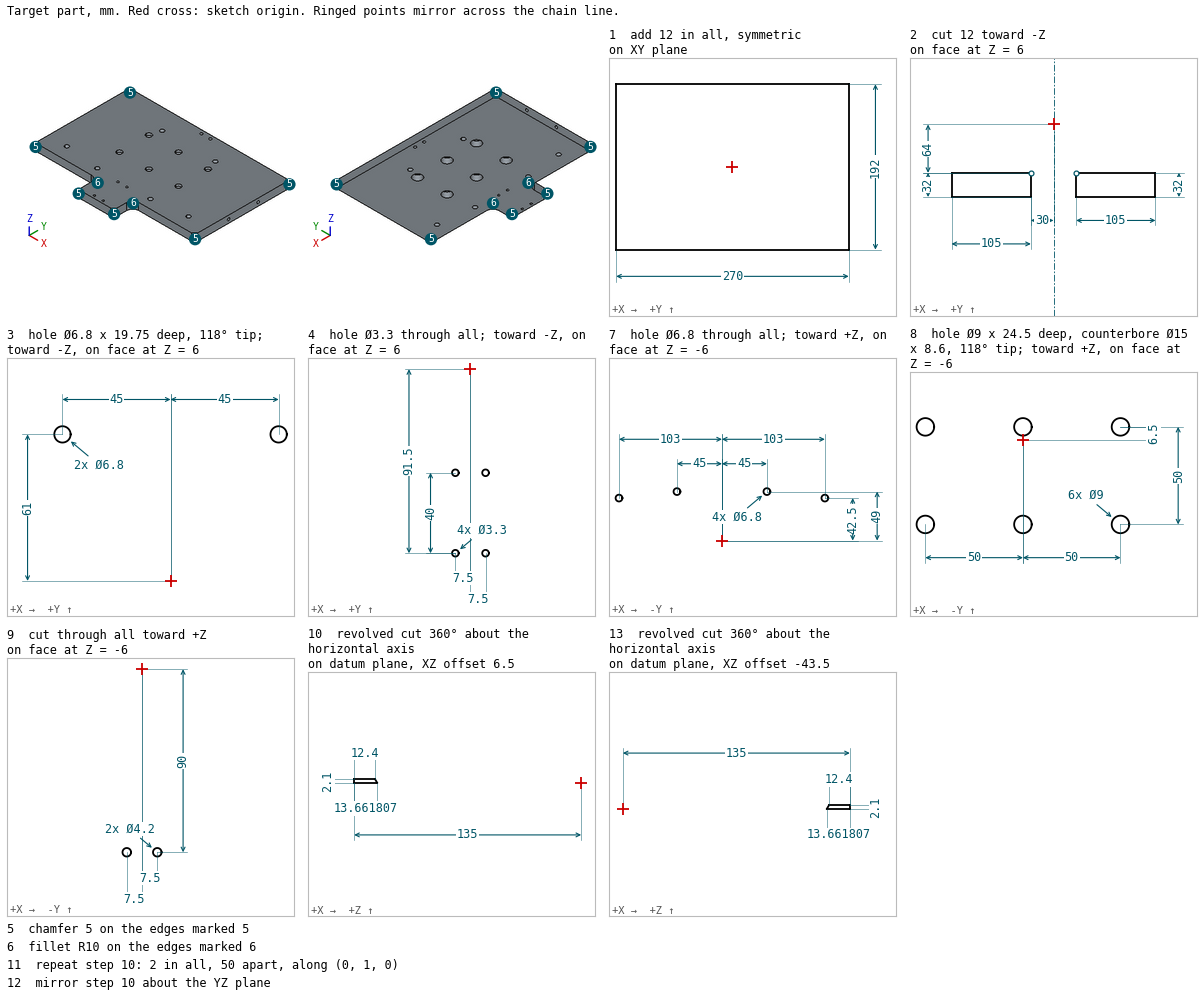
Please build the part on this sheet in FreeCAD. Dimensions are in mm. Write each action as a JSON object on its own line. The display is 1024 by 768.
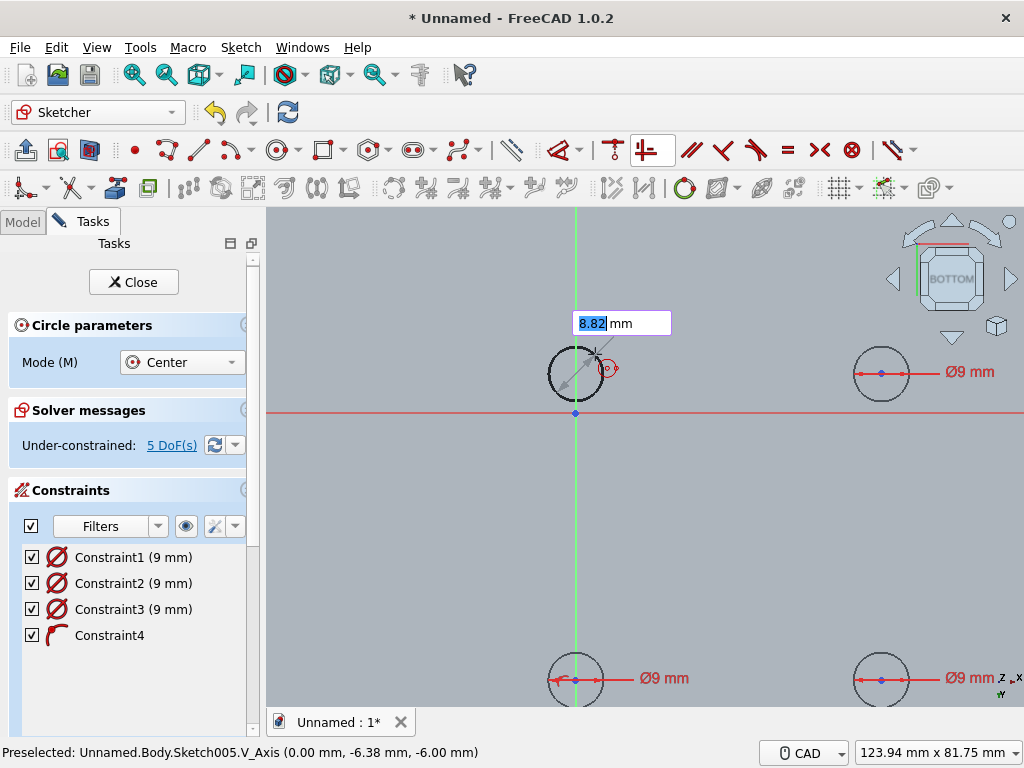
{"action": "type", "text": "9"}
{"action": "key", "text": "Return"}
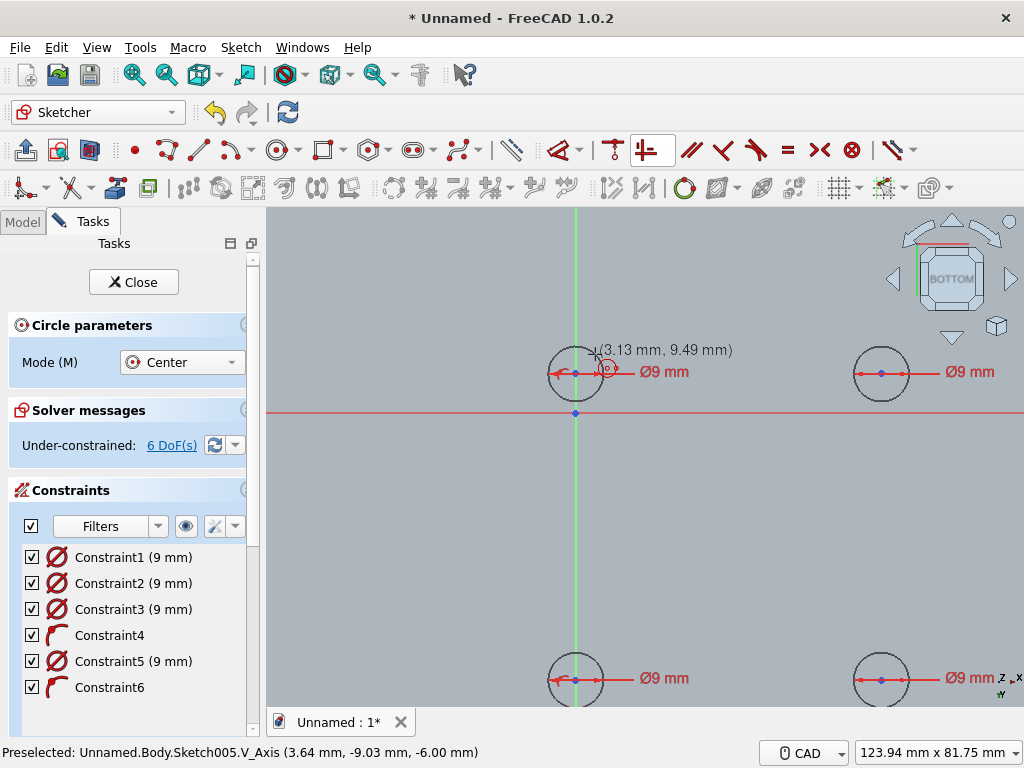
{"action": "scroll", "coordinate": [577, 373], "scroll_direction": "down", "scroll_amount": 3}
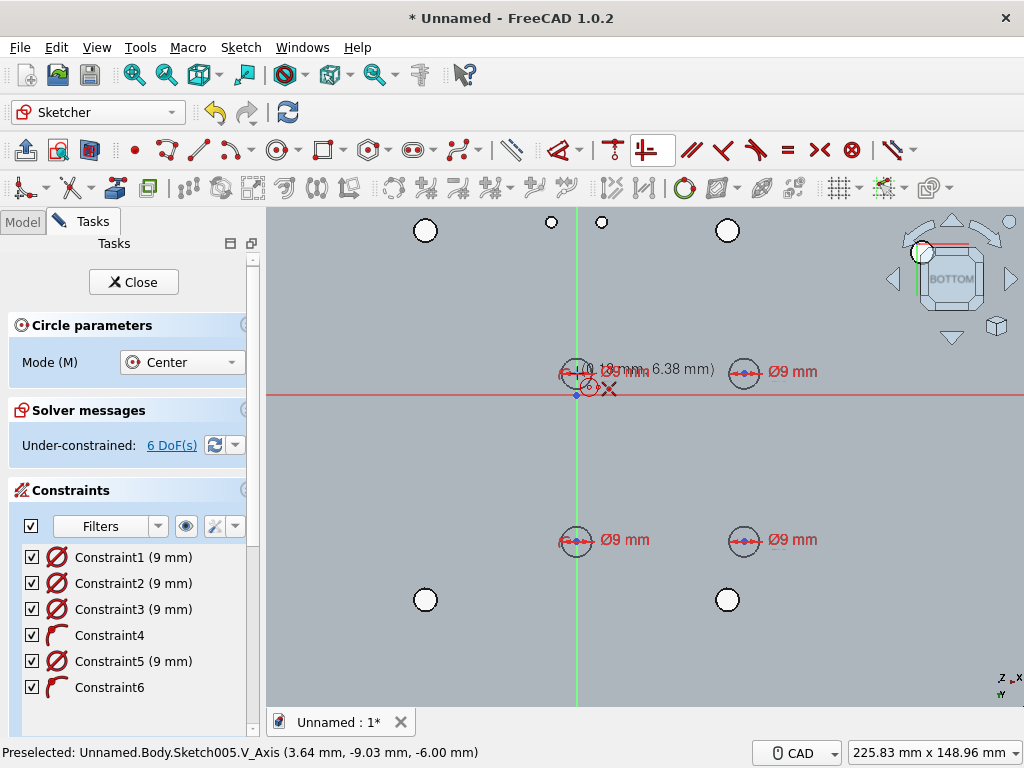
{"action": "scroll", "coordinate": [409, 541], "scroll_direction": "up", "scroll_amount": 3}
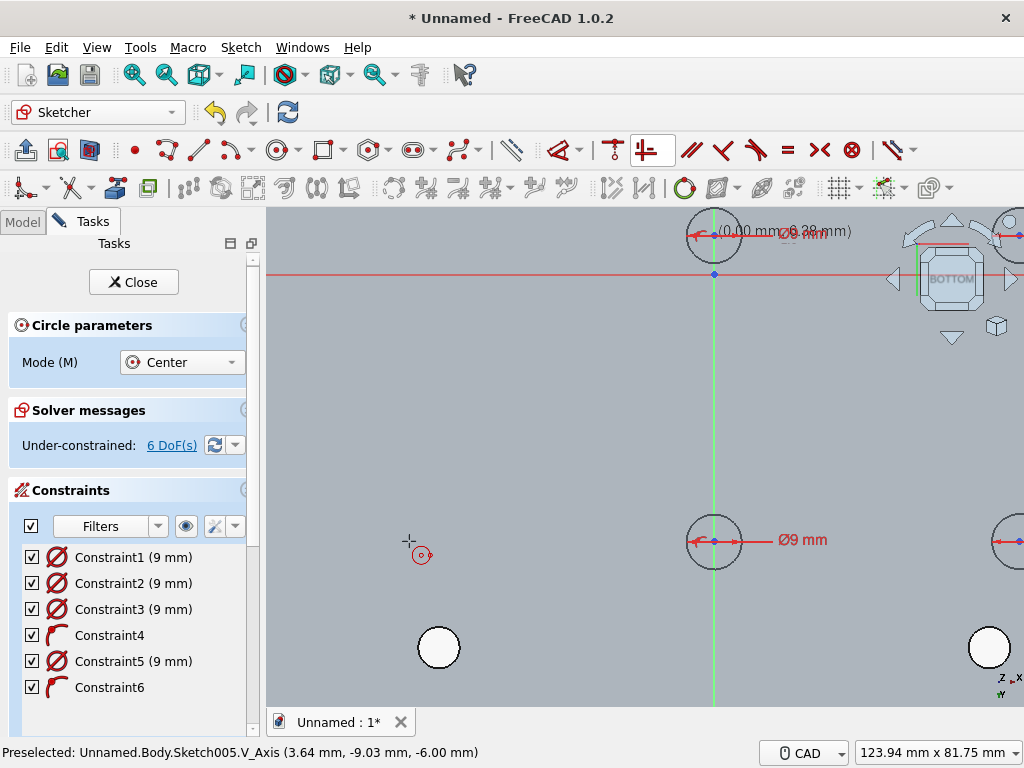
{"action": "left_click", "coordinate": [408, 541]}
{"action": "mouse_move", "coordinate": [428, 521]}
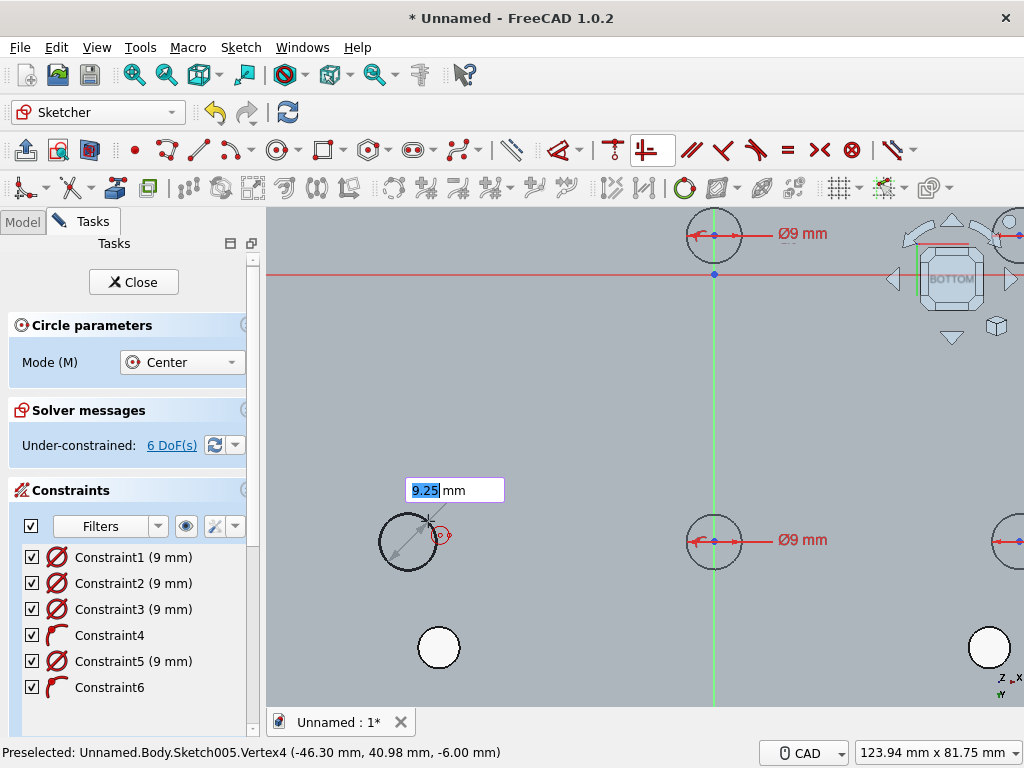
{"action": "type", "text": "9"}
{"action": "key", "text": "Return"}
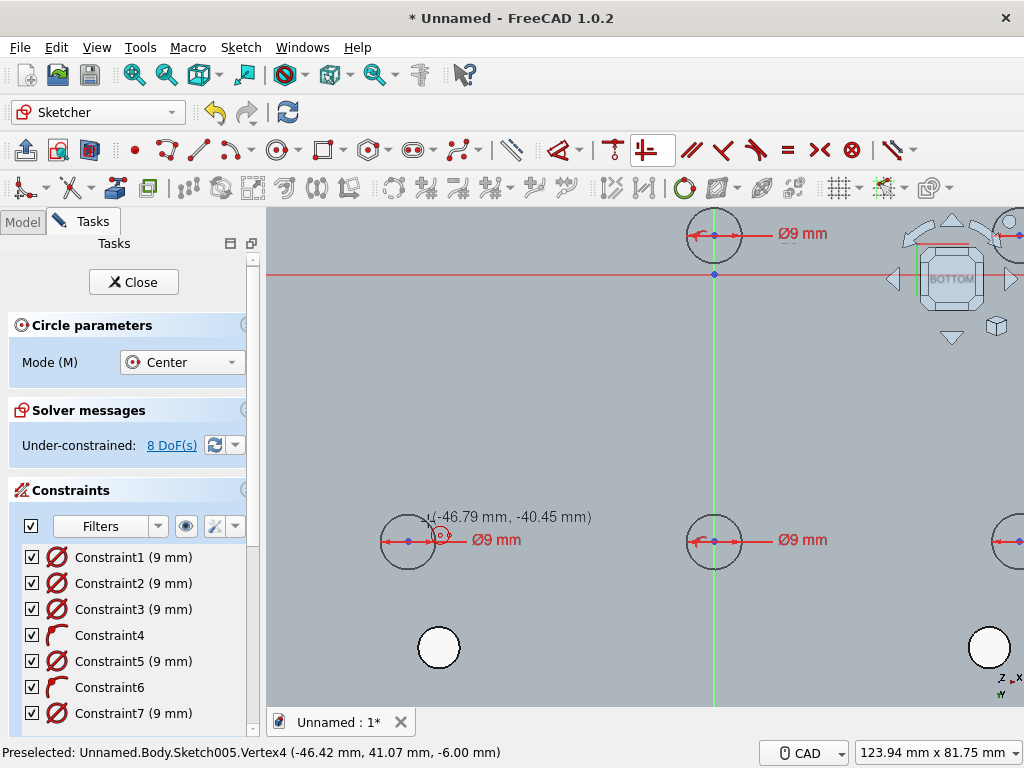
{"action": "scroll", "coordinate": [409, 541], "scroll_direction": "down", "scroll_amount": 3}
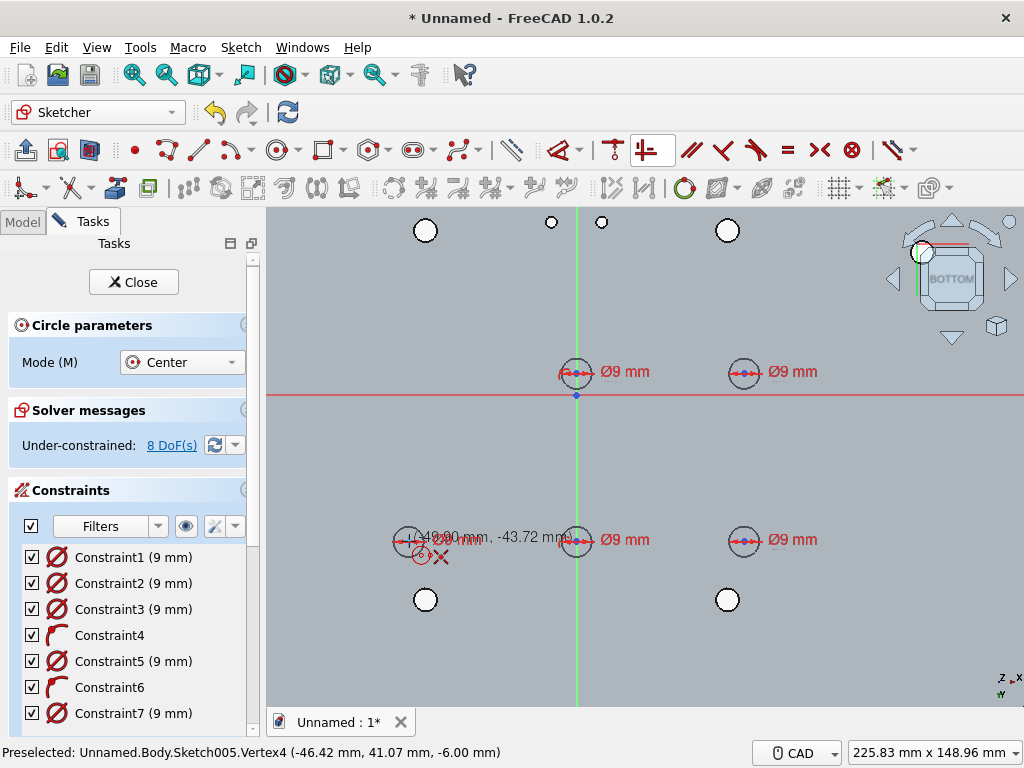
{"action": "scroll", "coordinate": [409, 373], "scroll_direction": "up", "scroll_amount": 3}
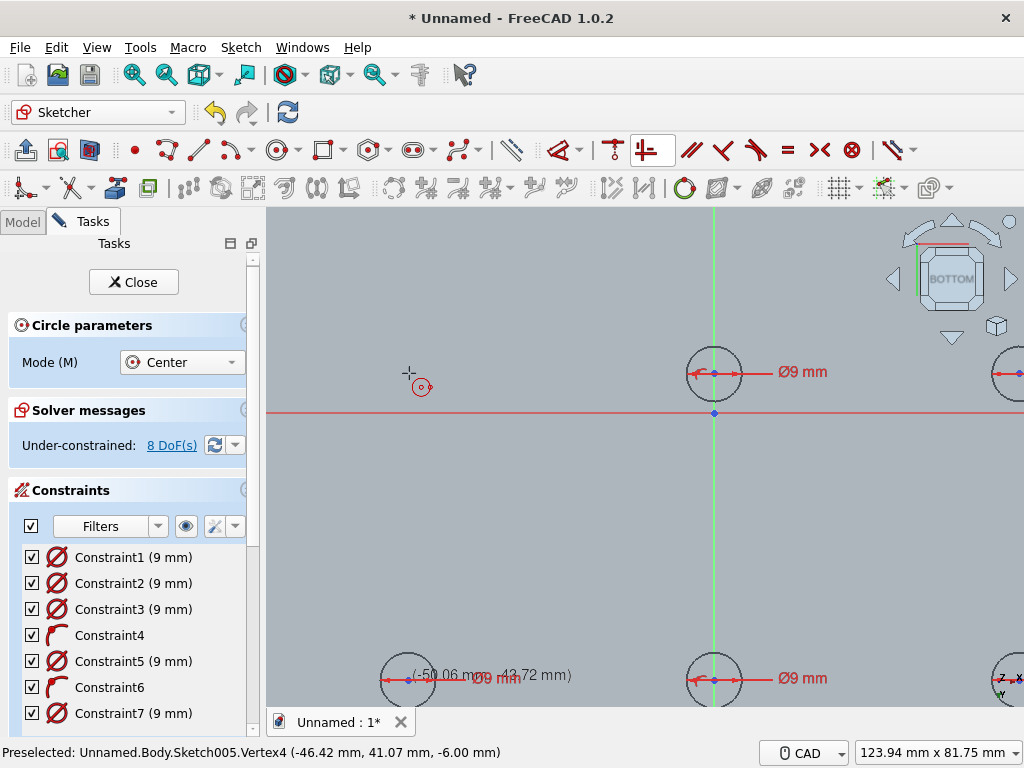
{"action": "left_click", "coordinate": [408, 373]}
{"action": "mouse_move", "coordinate": [428, 354]}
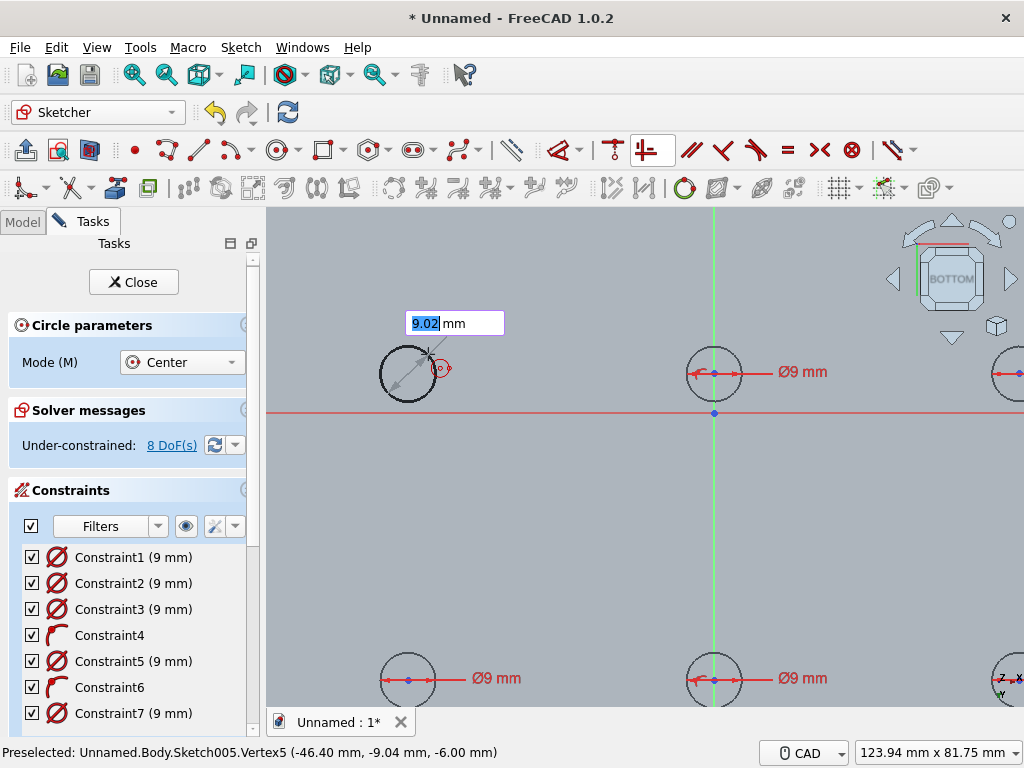
{"action": "type", "text": "9"}
{"action": "key", "text": "Return"}
{"action": "key", "text": "Escape"}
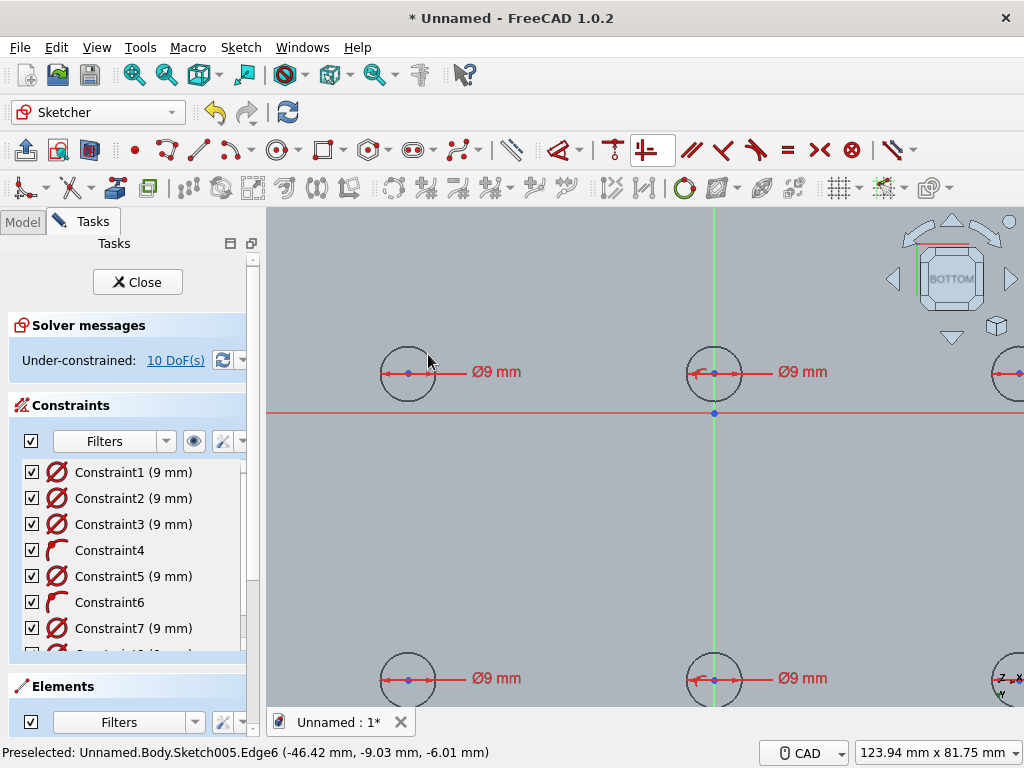
{"action": "scroll", "coordinate": [409, 373], "scroll_direction": "down", "scroll_amount": 3}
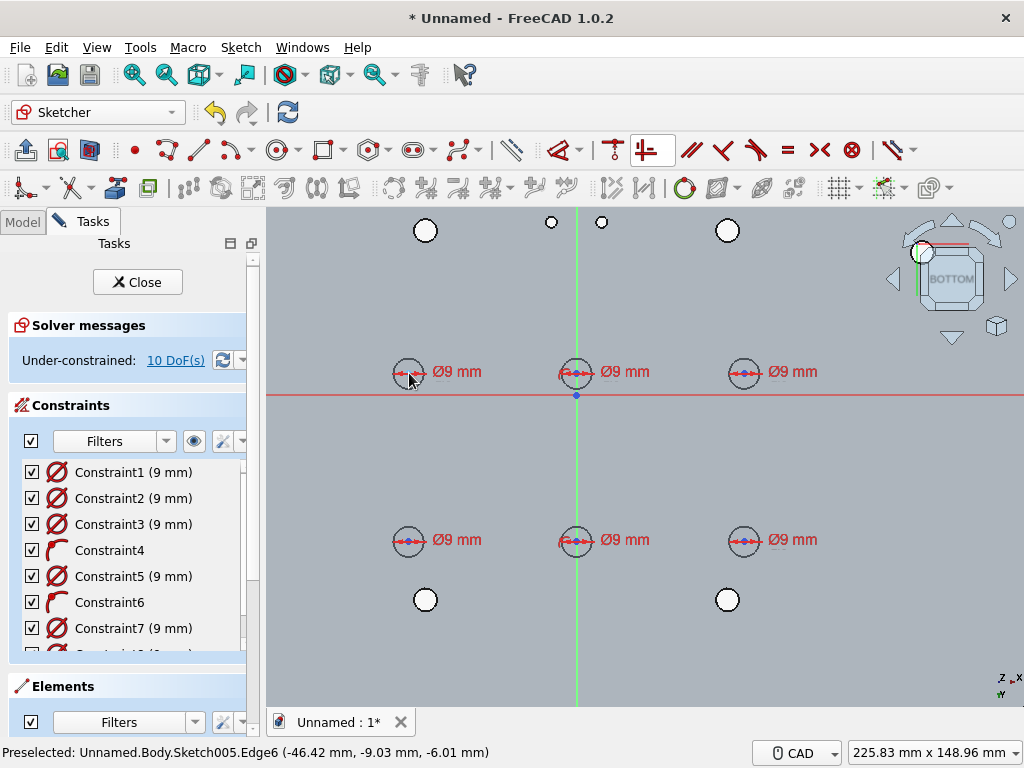
{"action": "left_click", "coordinate": [744, 542]}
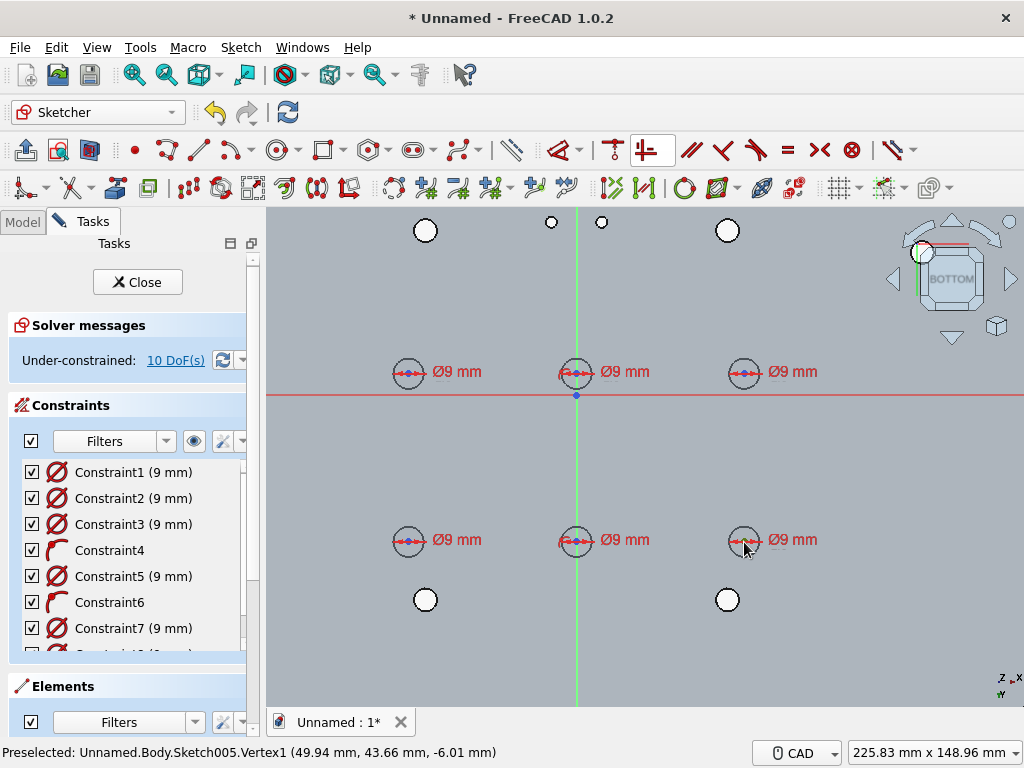
{"action": "left_click", "coordinate": [744, 374]}